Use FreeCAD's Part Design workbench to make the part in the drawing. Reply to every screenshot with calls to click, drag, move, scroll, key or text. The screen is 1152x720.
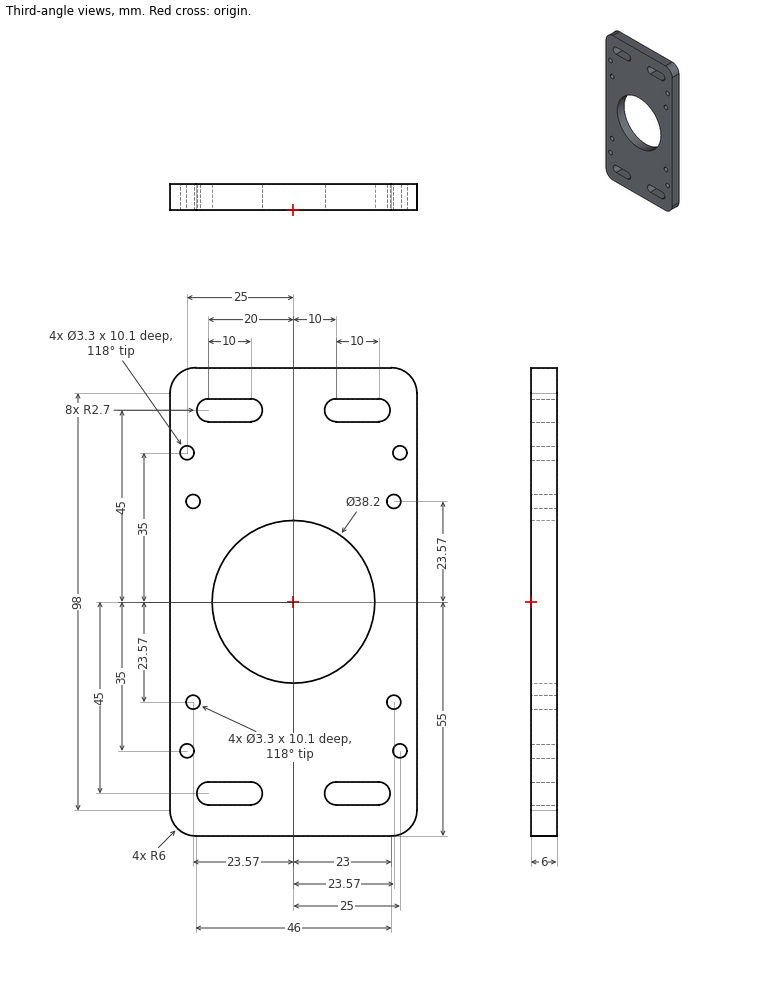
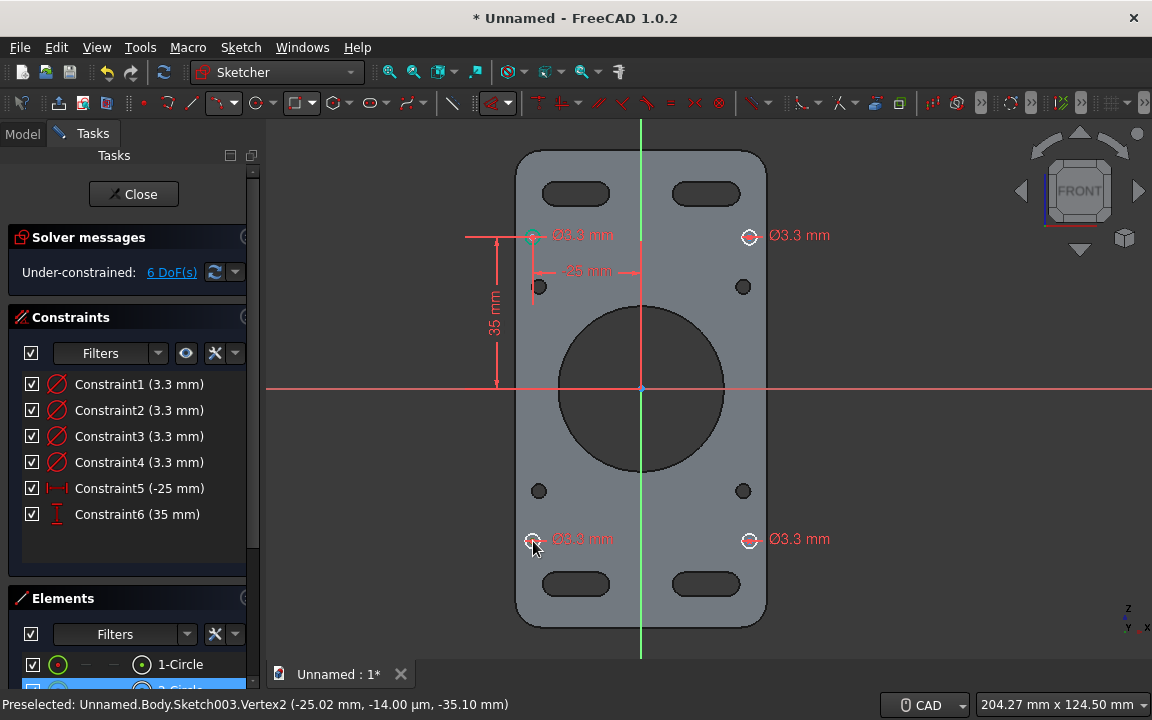
click(510, 104)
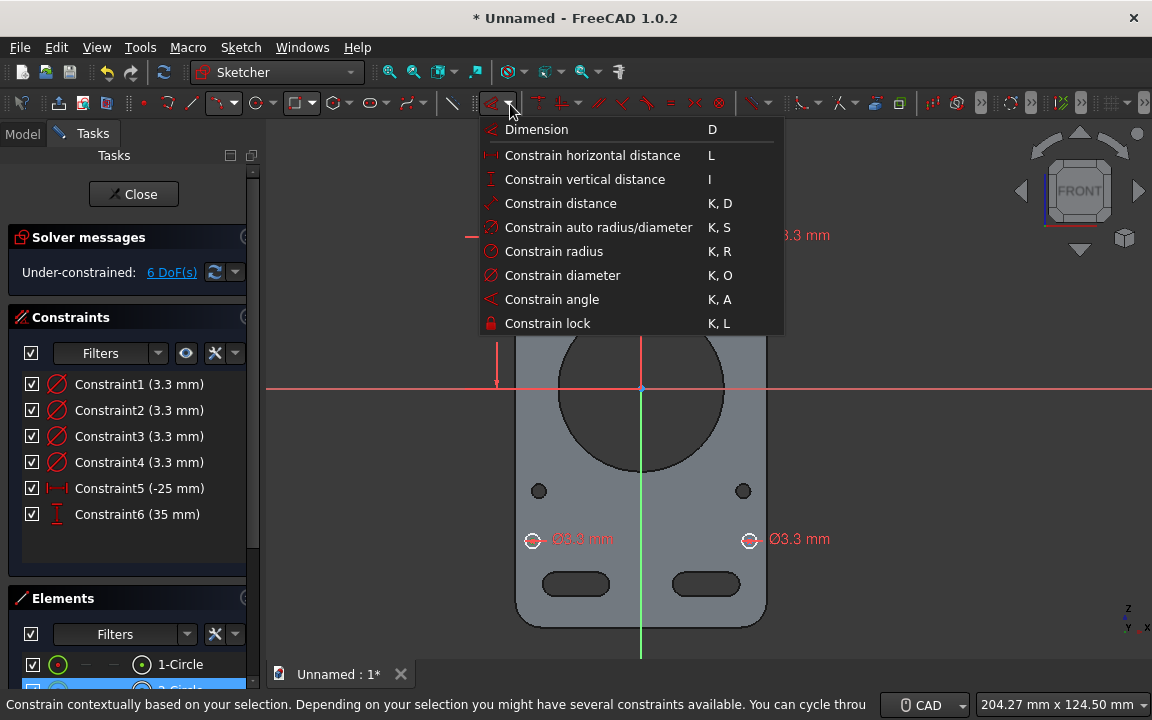
click(632, 155)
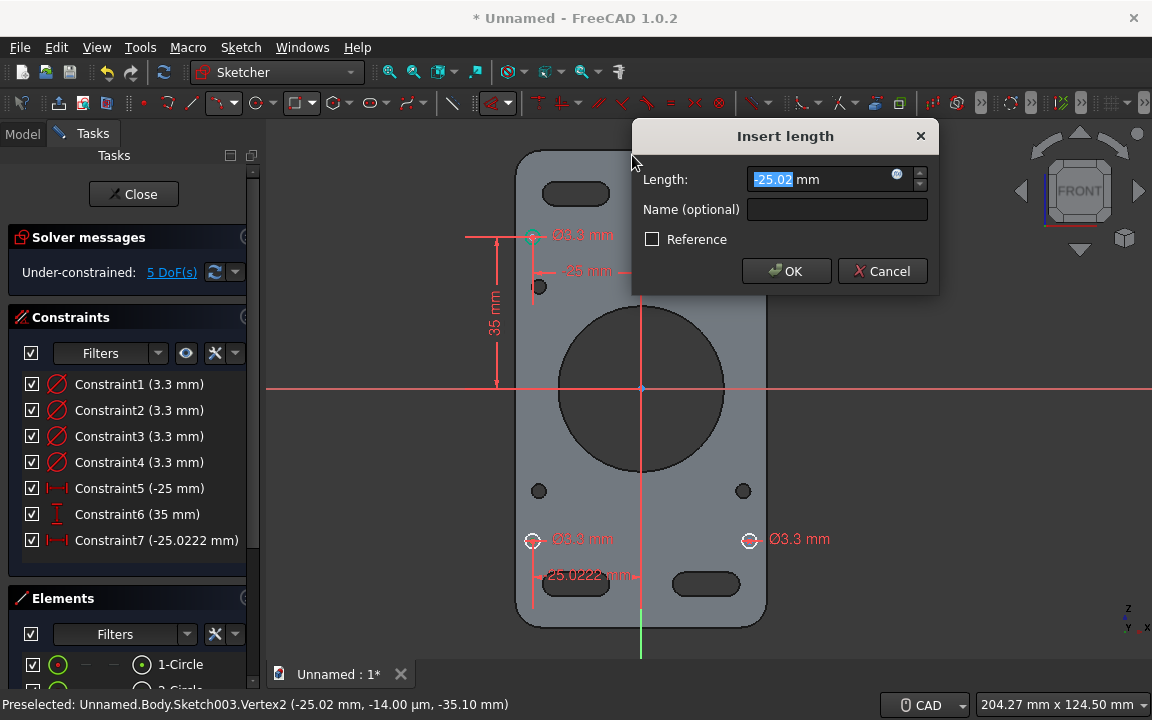
text(-25)
key(Return)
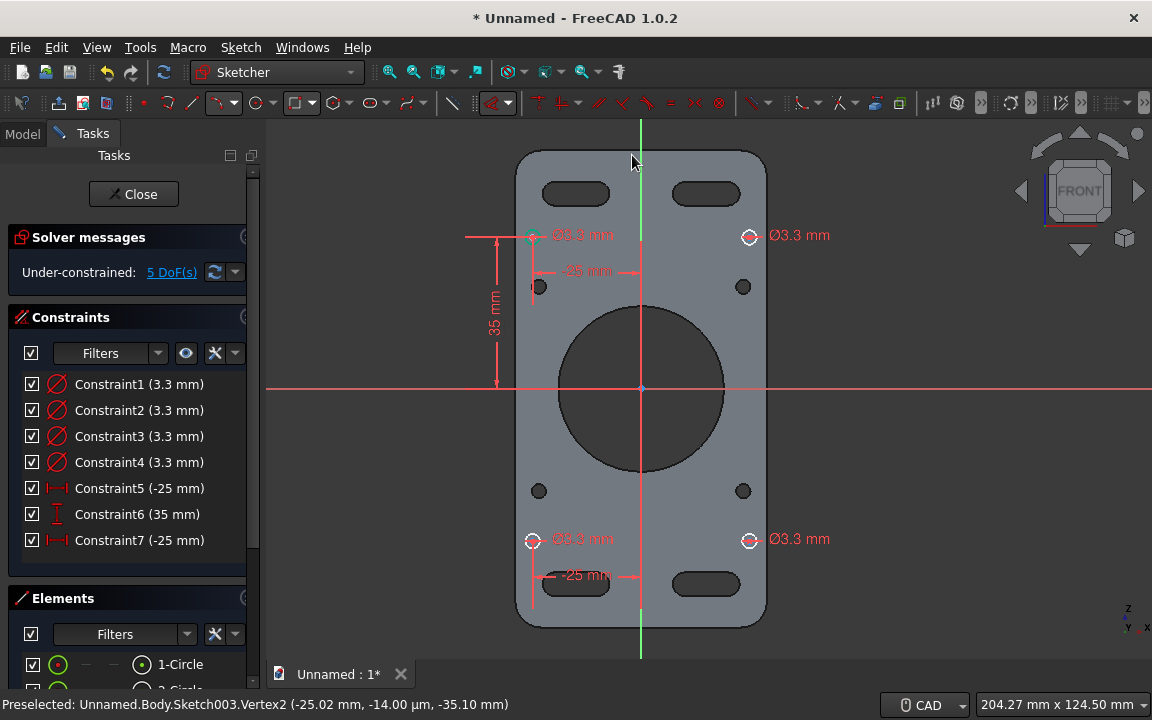
click(533, 541)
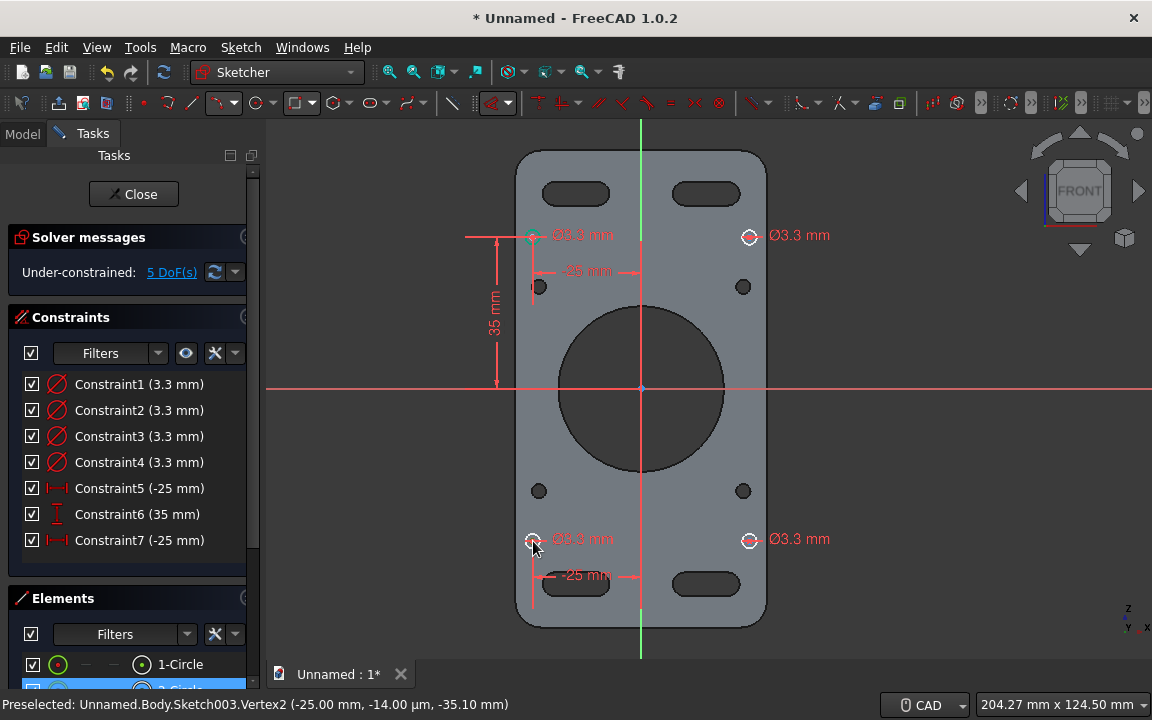
key(i)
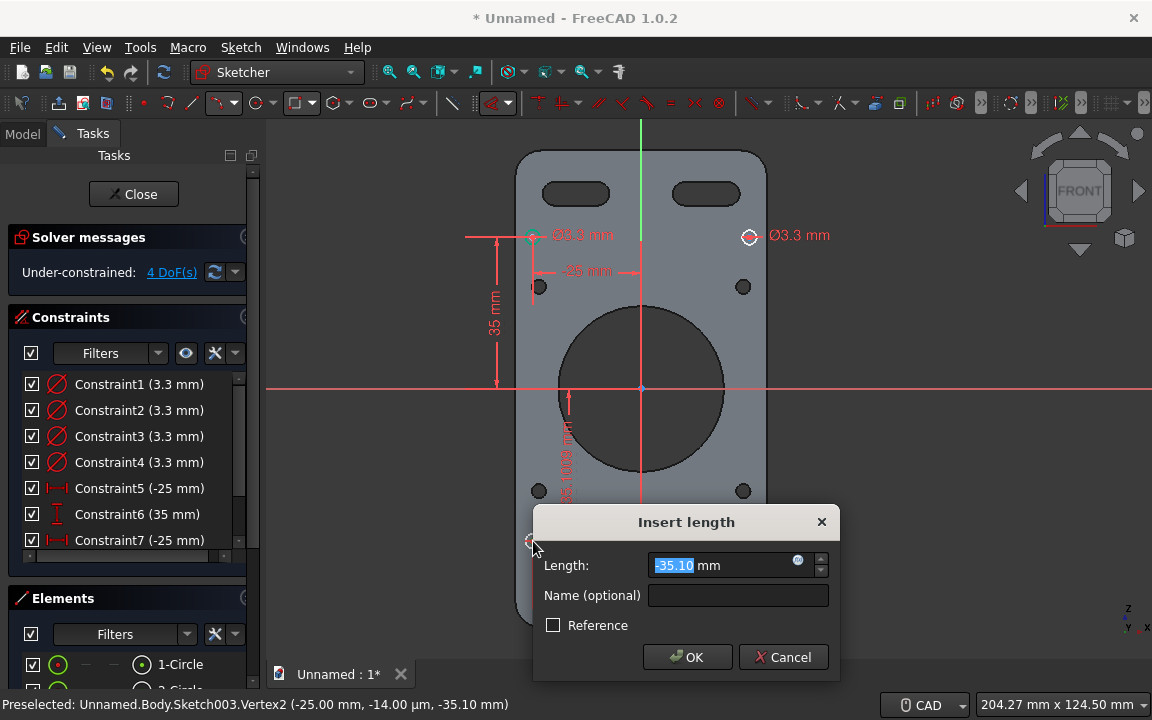
text(-35)
key(Return)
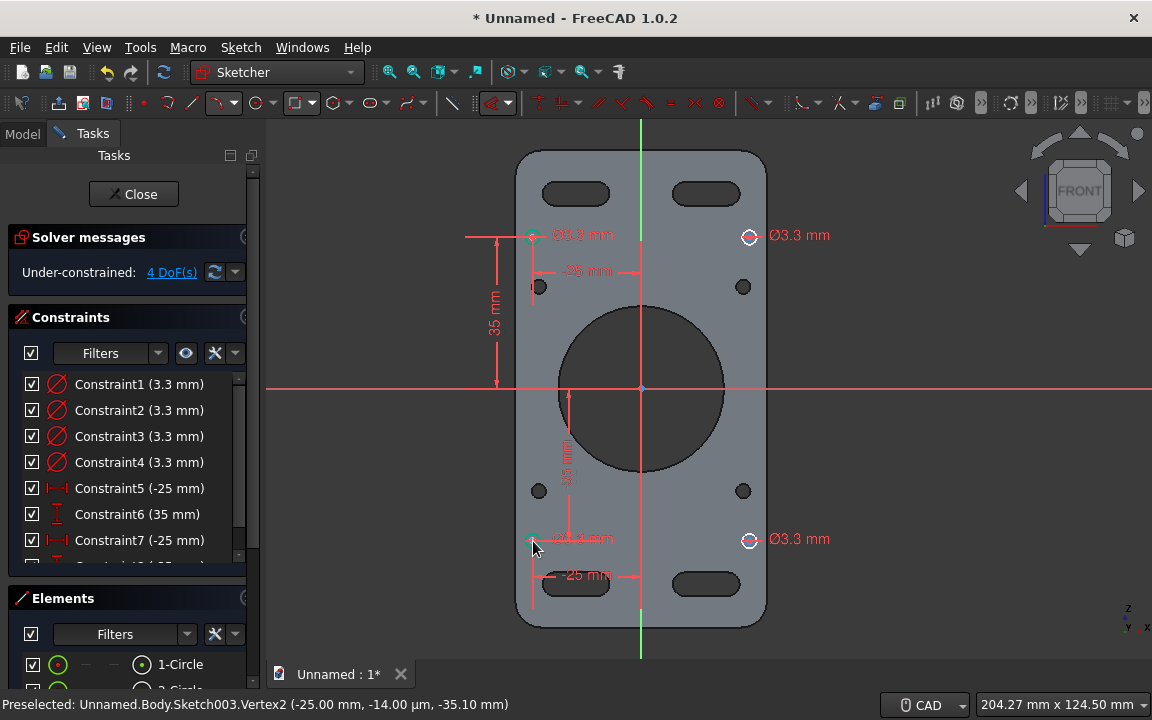
click(749, 541)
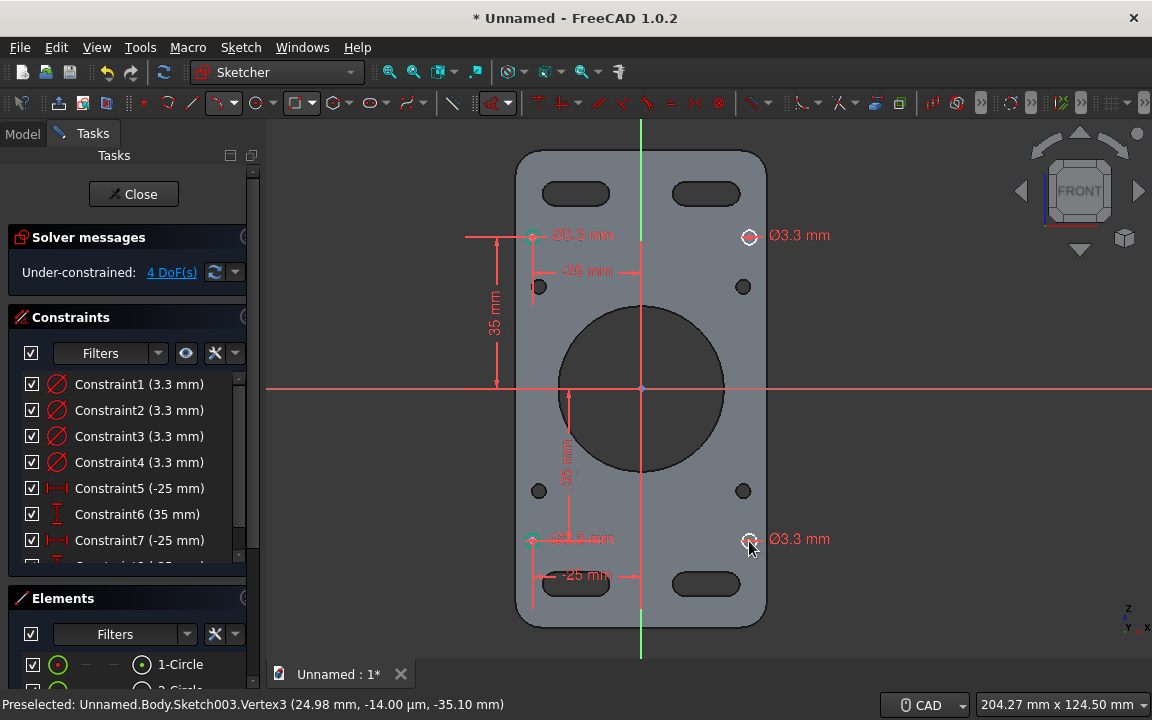
click(510, 104)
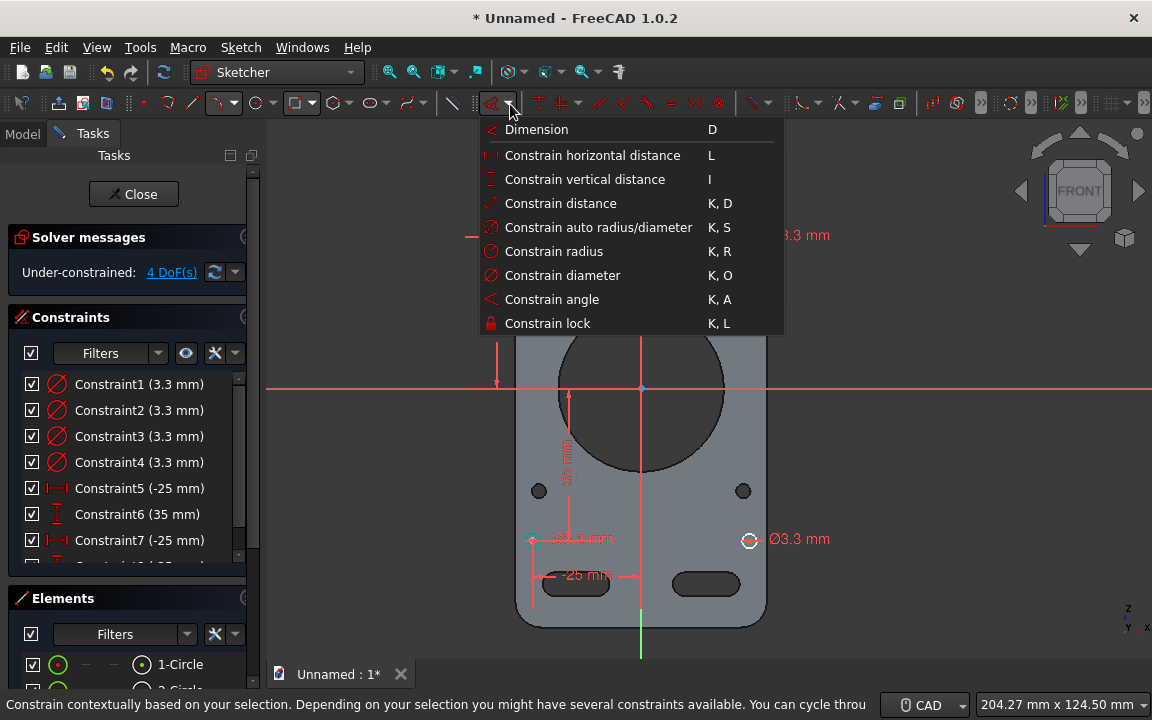
click(632, 155)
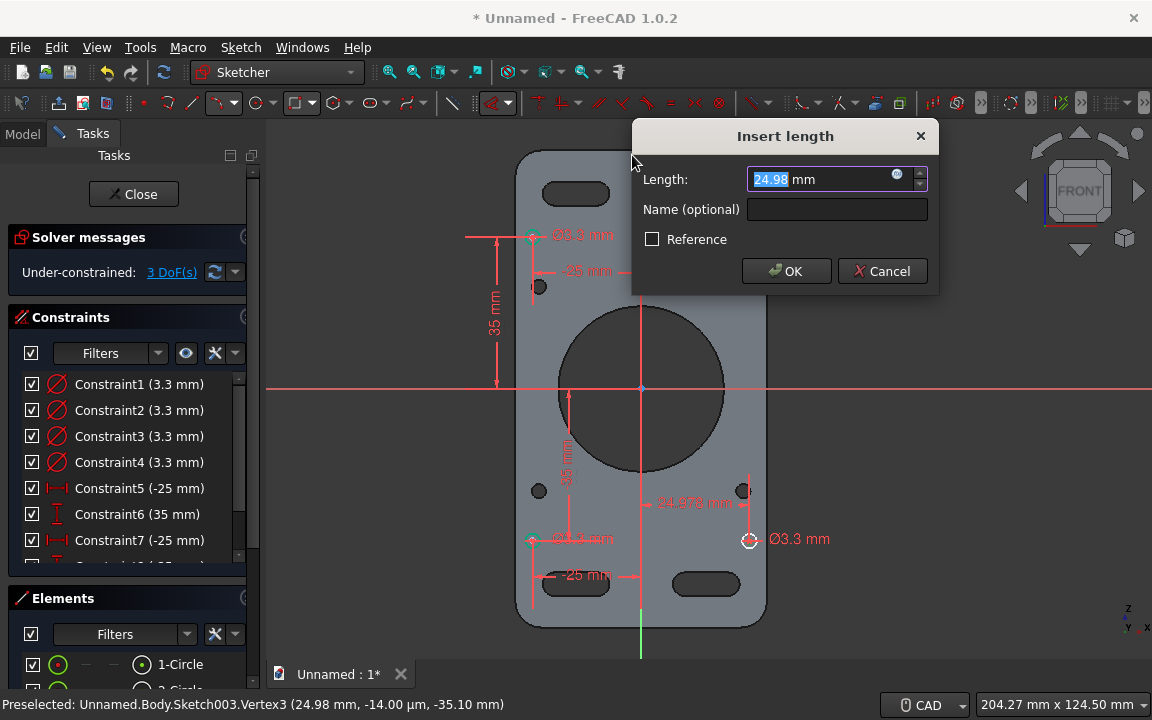
text(25)
key(Return)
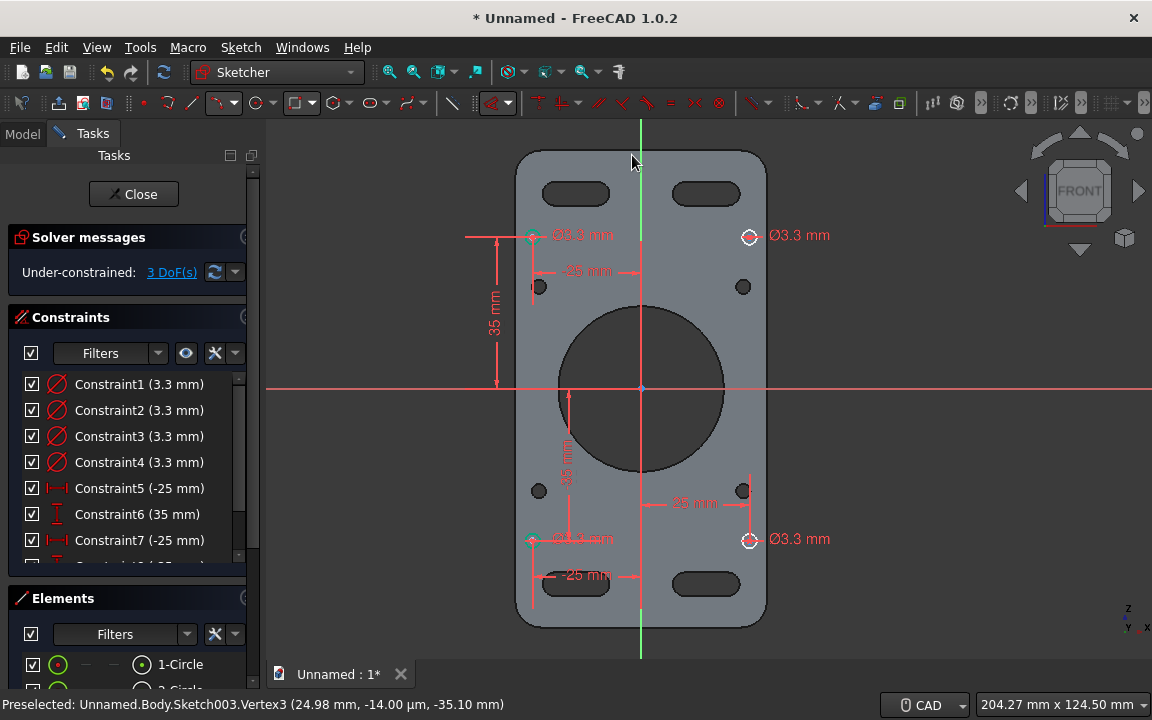
click(750, 541)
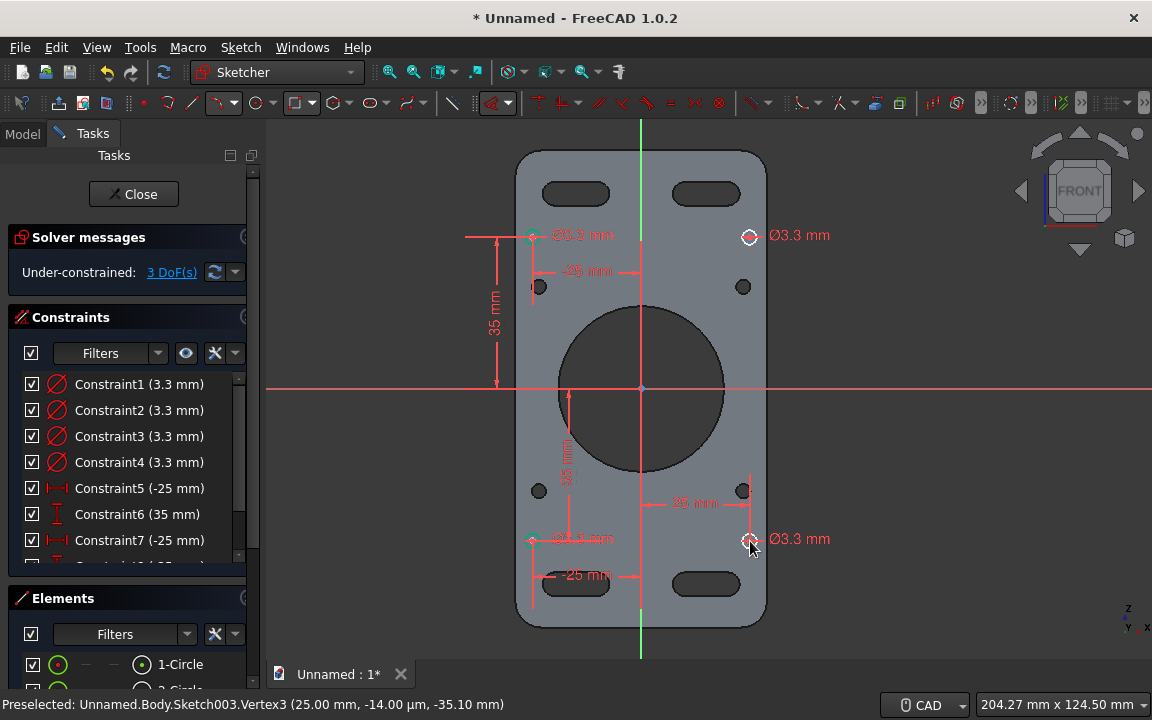
click(510, 104)